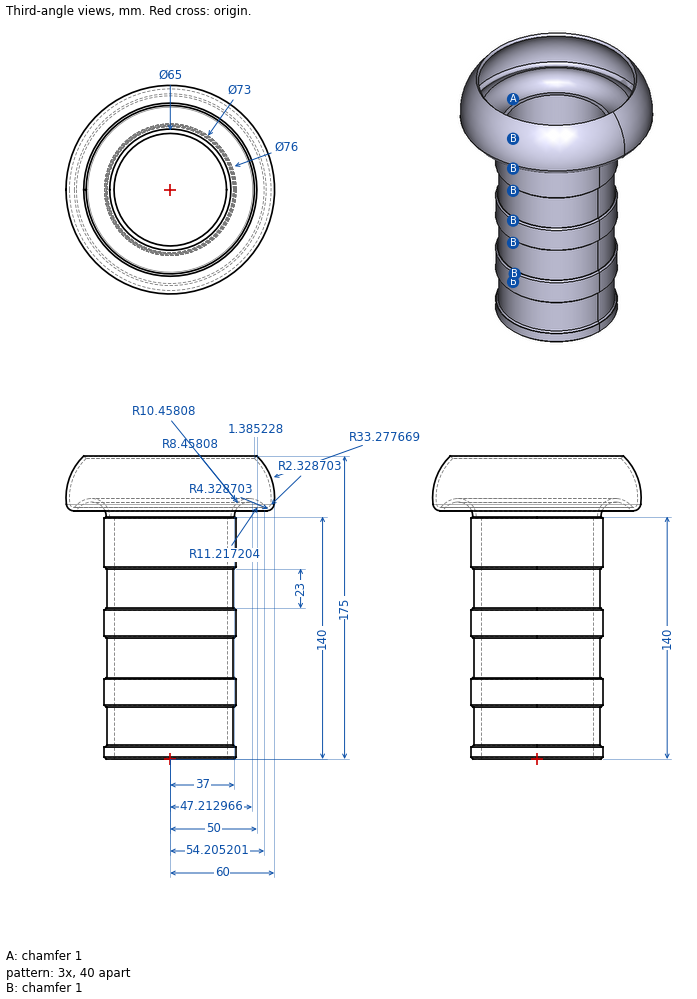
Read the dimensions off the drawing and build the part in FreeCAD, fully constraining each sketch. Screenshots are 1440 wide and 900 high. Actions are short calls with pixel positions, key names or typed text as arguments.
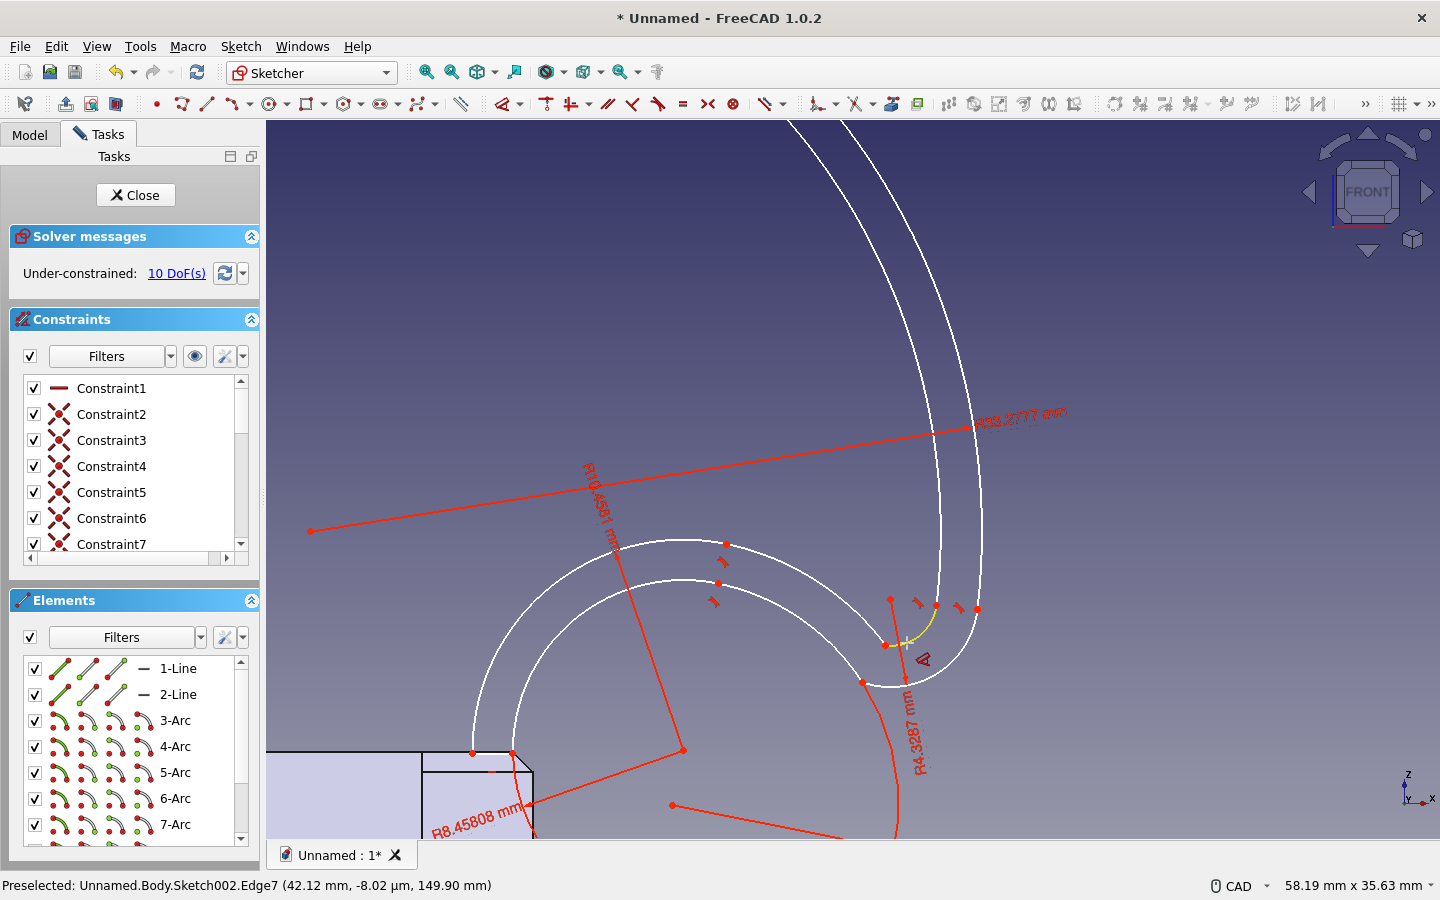
click(907, 643)
click(964, 572)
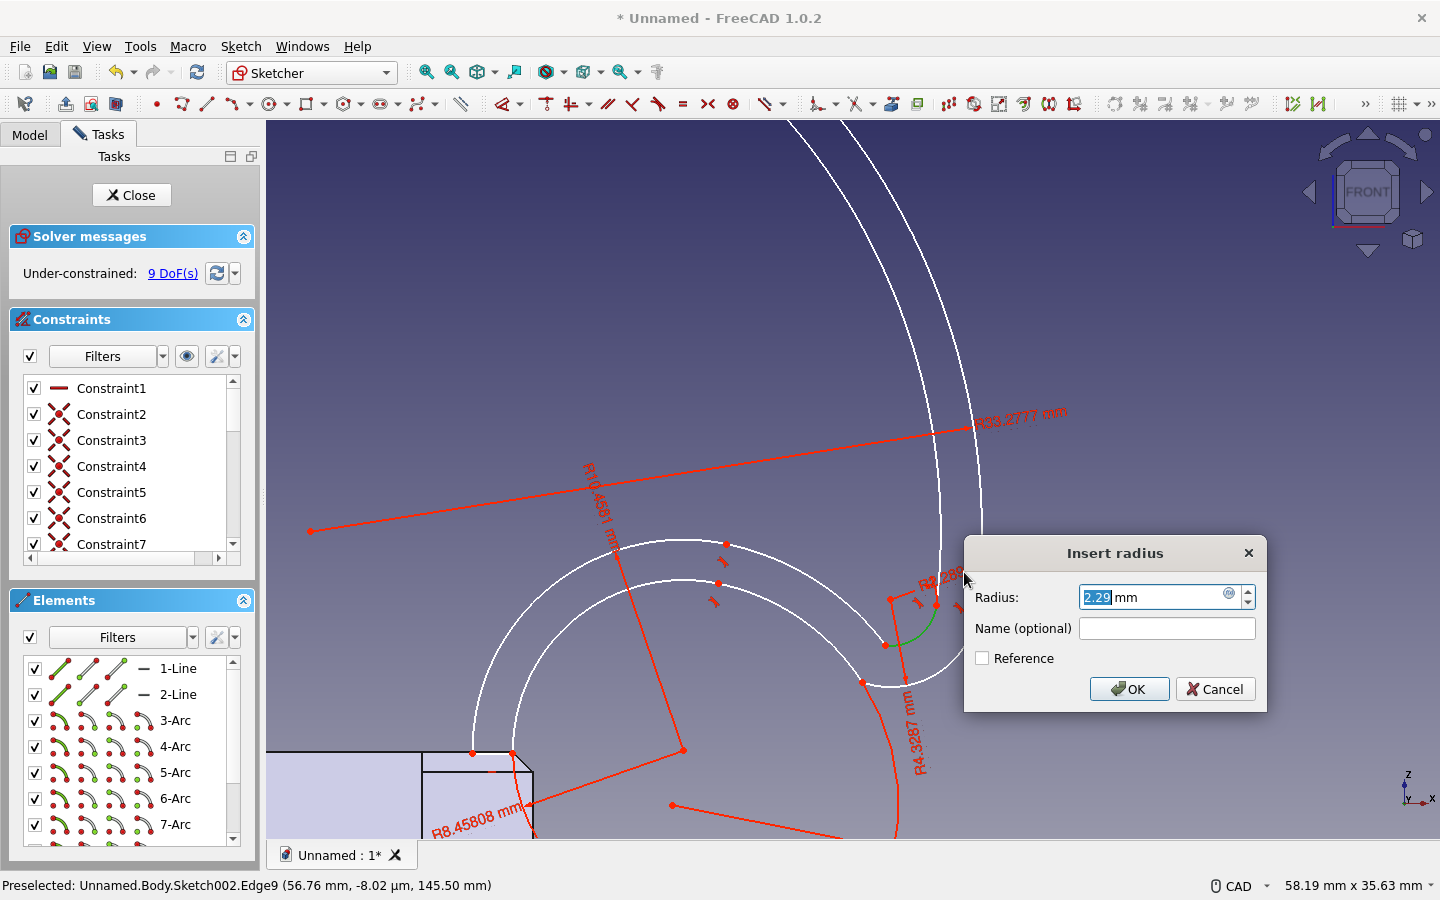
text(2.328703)
key(Return)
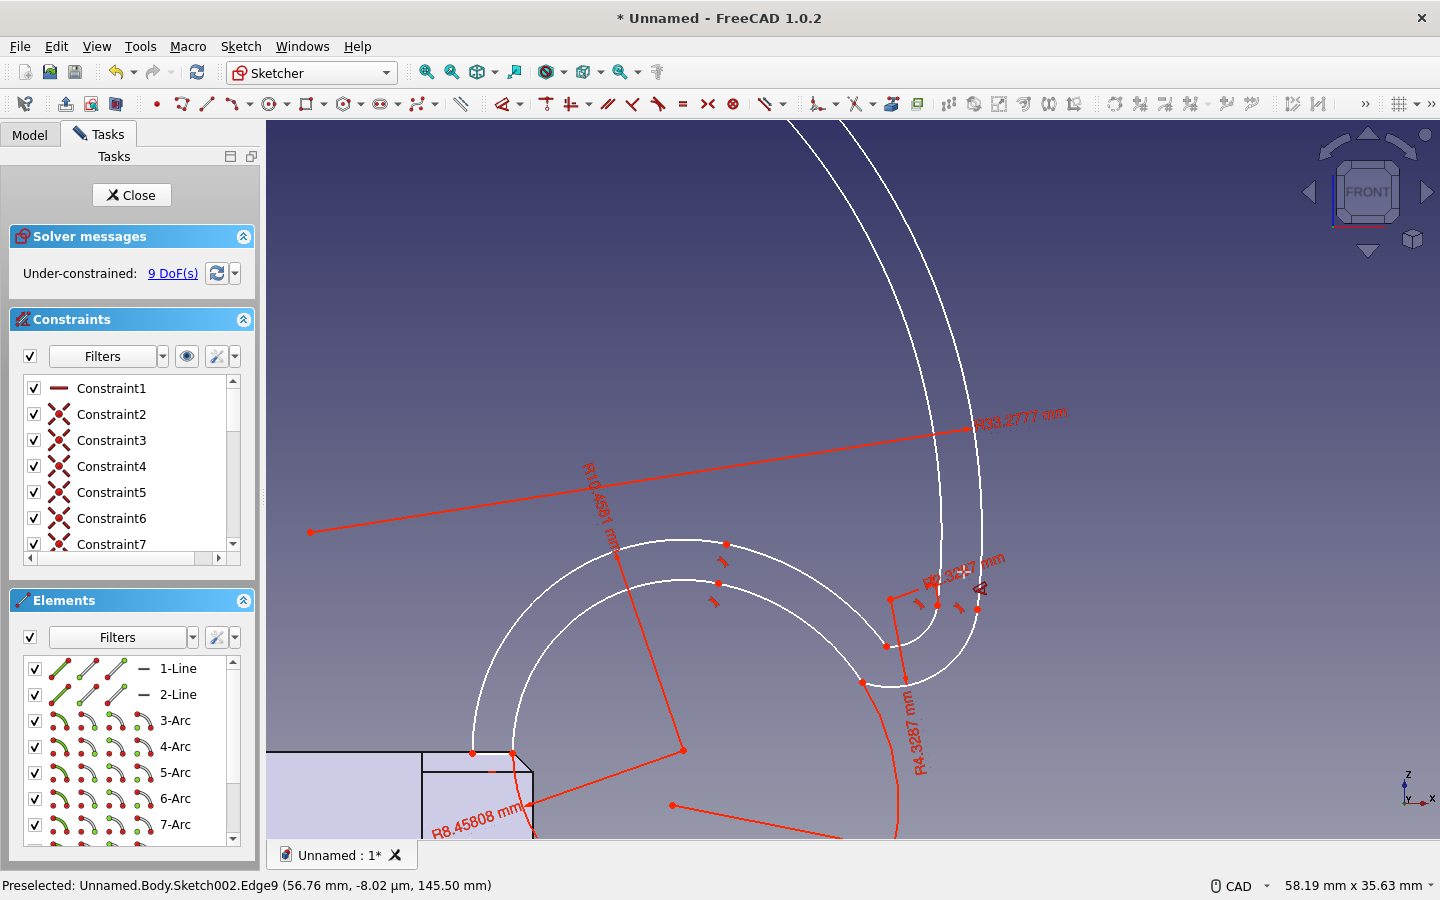
scroll(907, 643, down, 2)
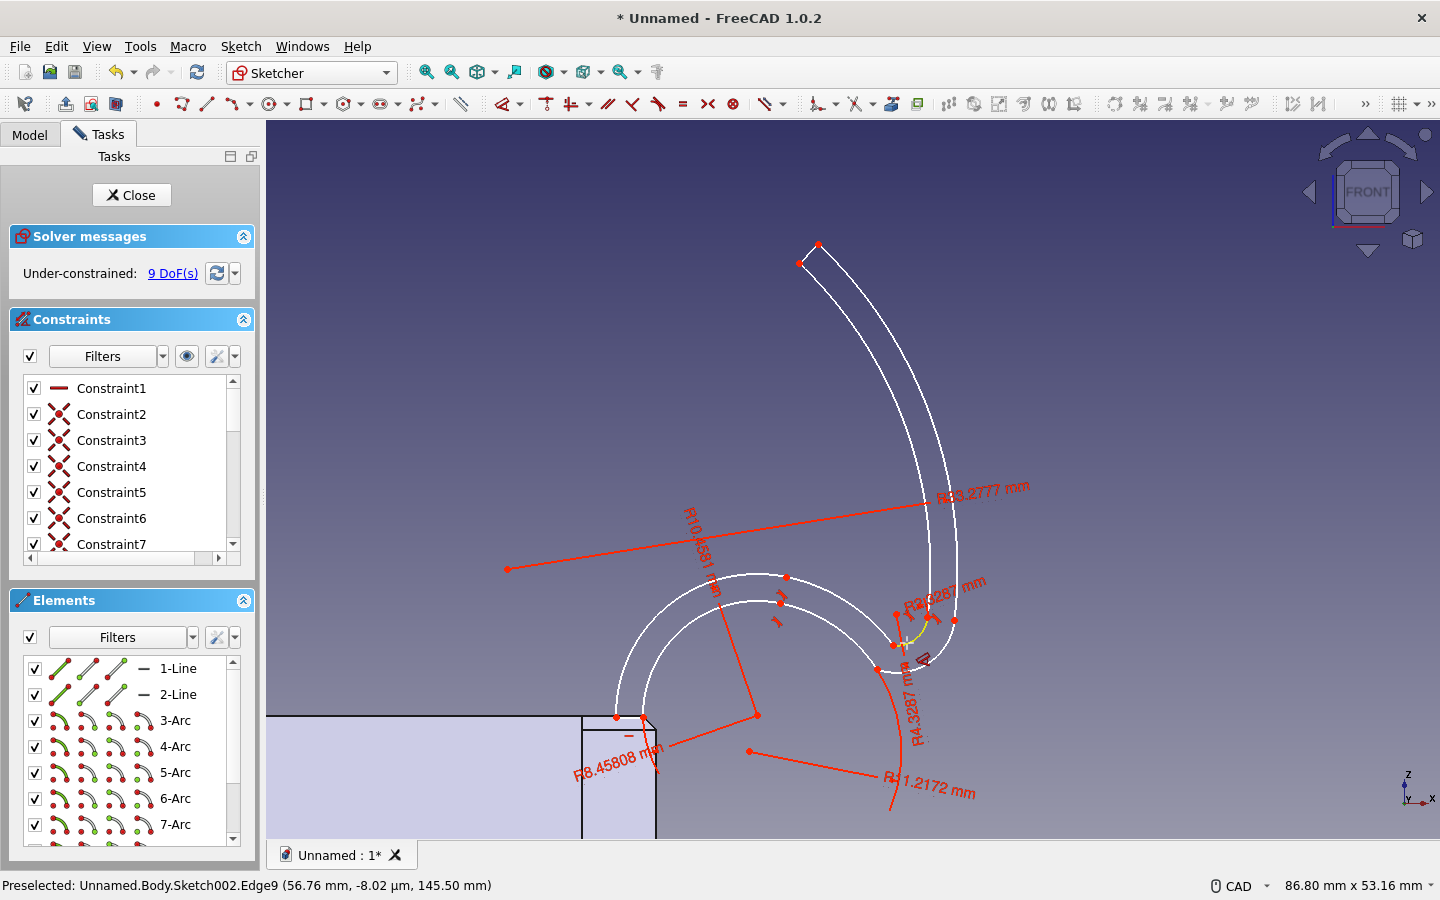
click(819, 244)
click(556, 210)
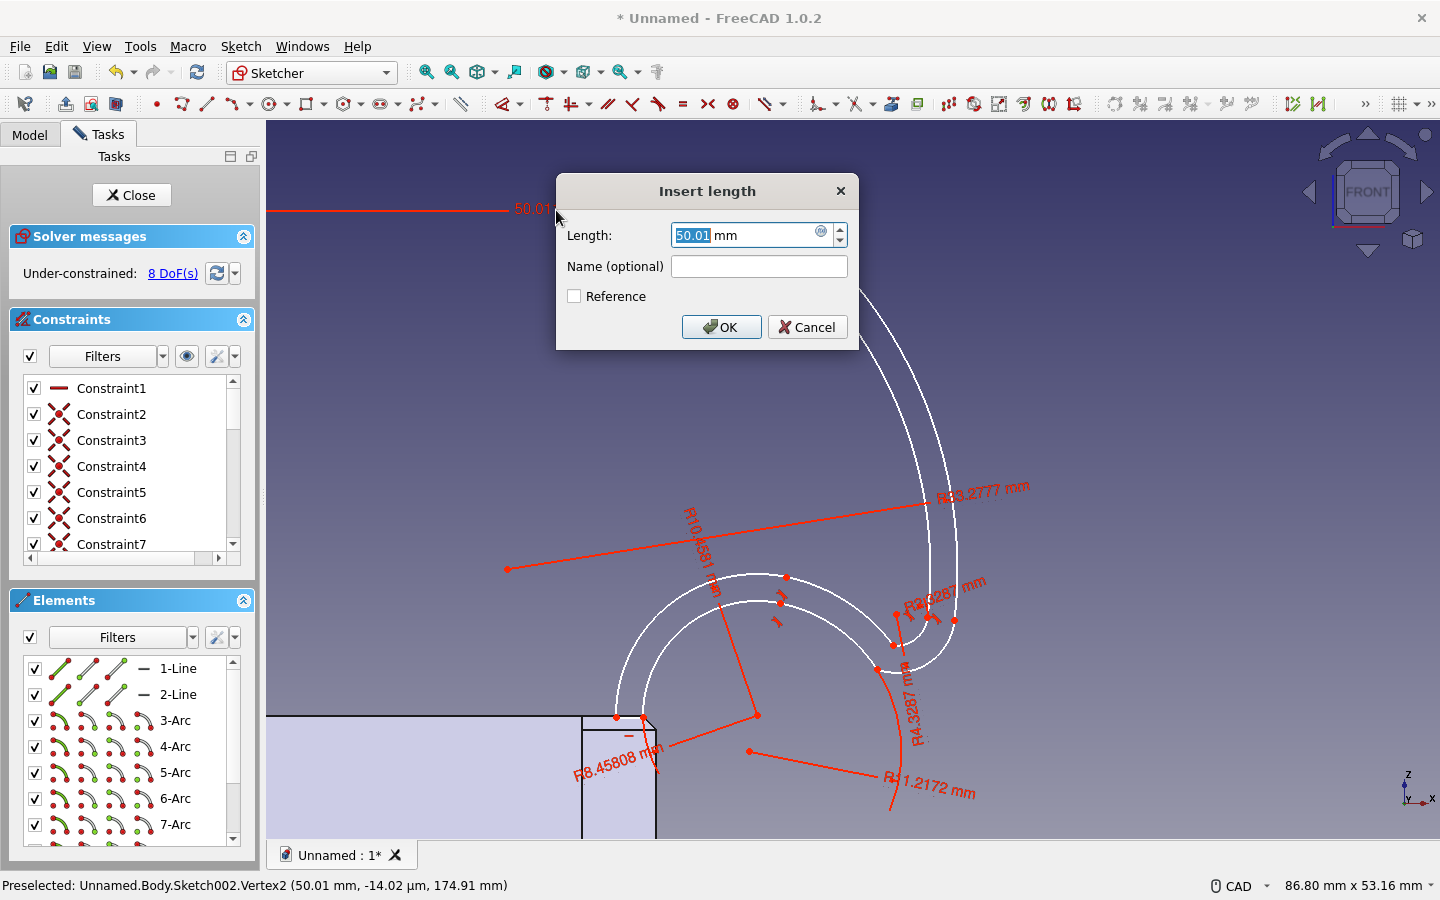
text(50)
key(Return)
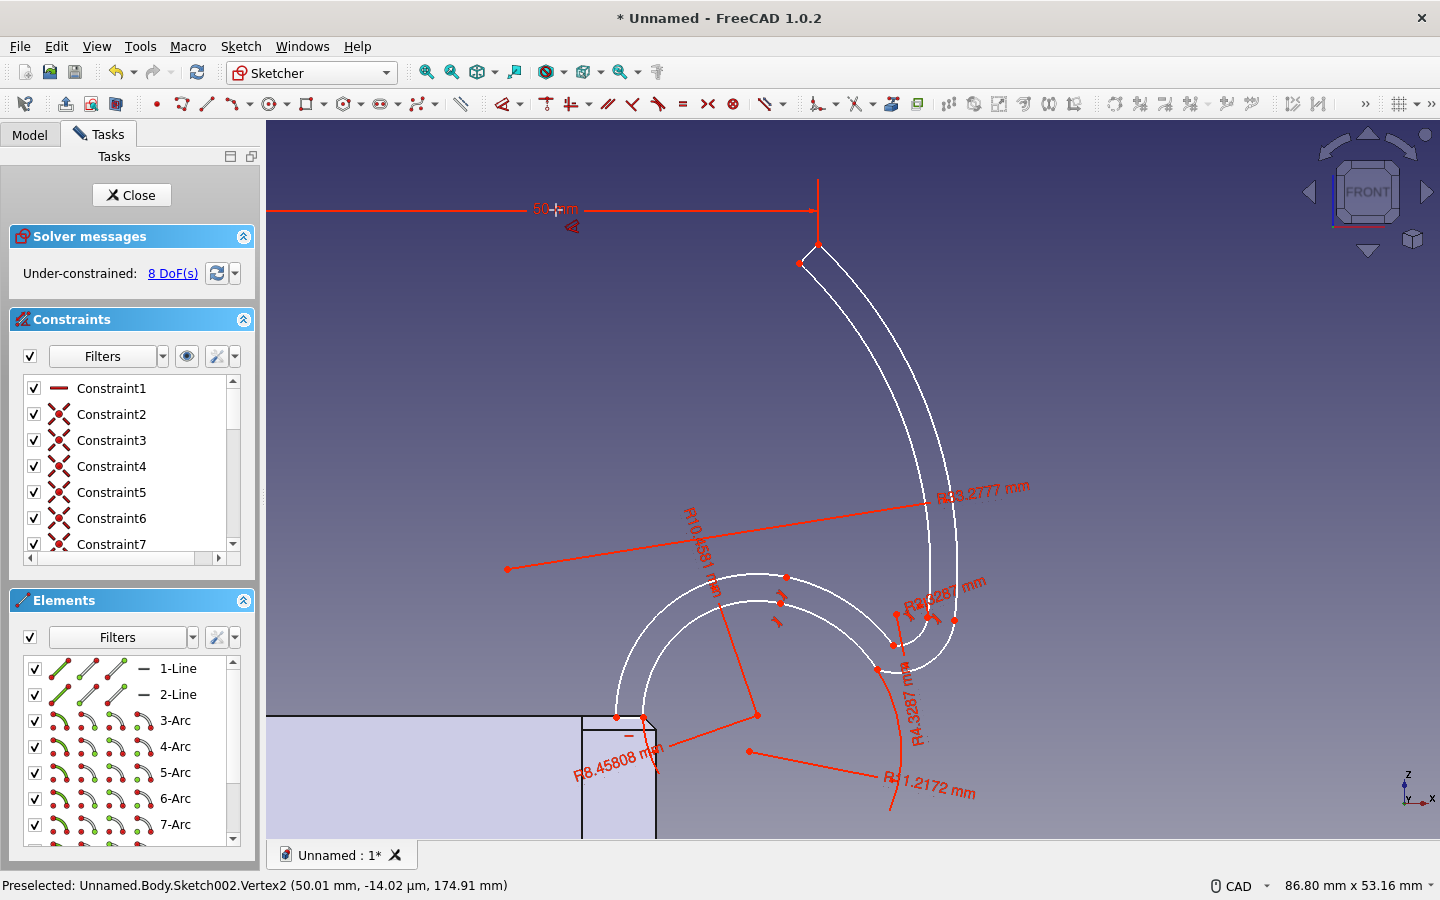
click(643, 718)
click(469, 684)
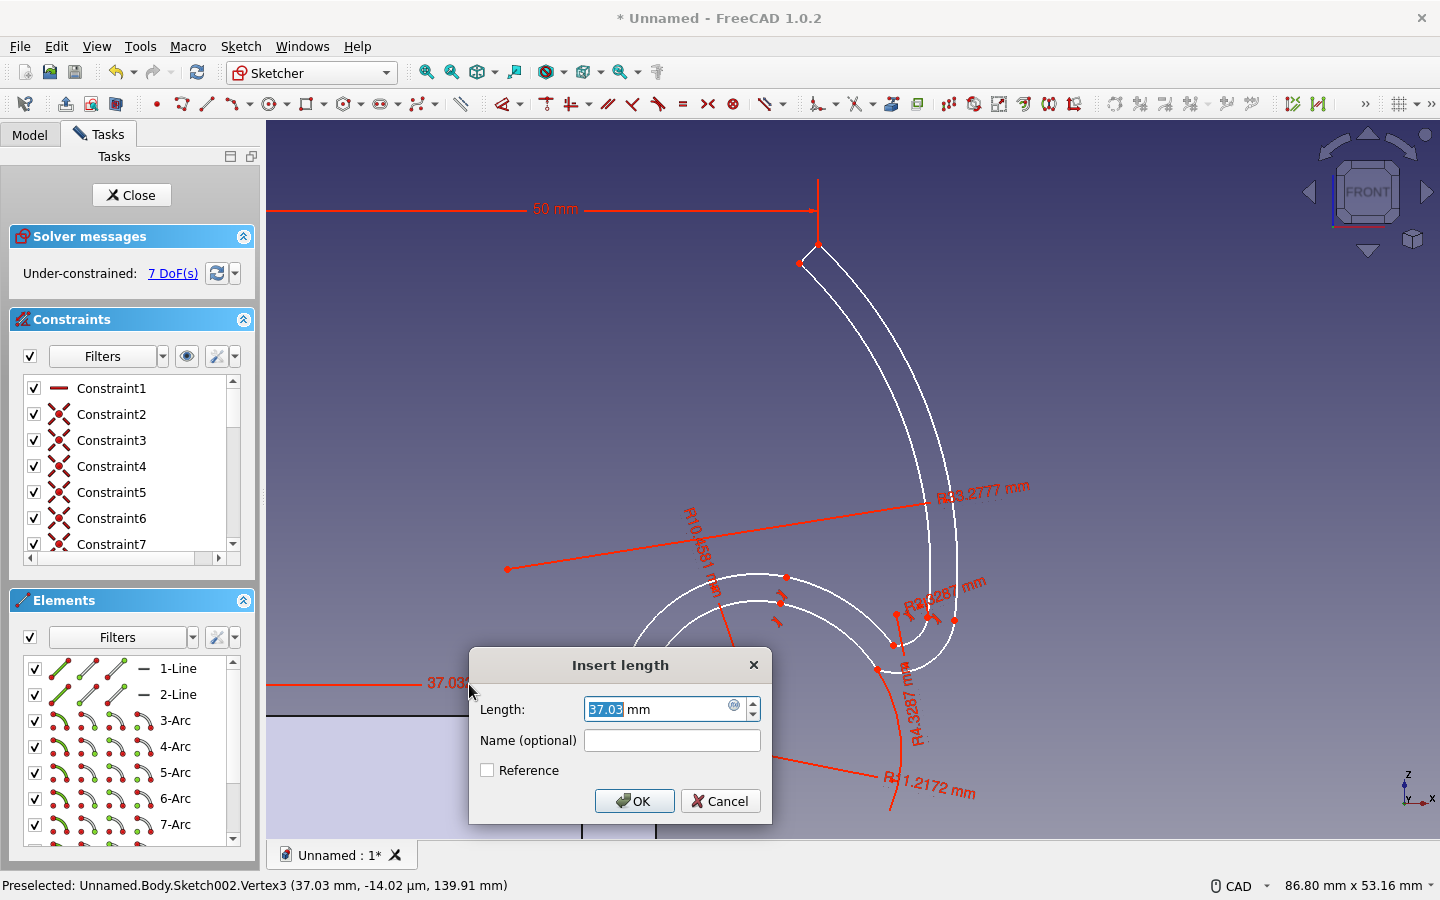
text(37)
key(Return)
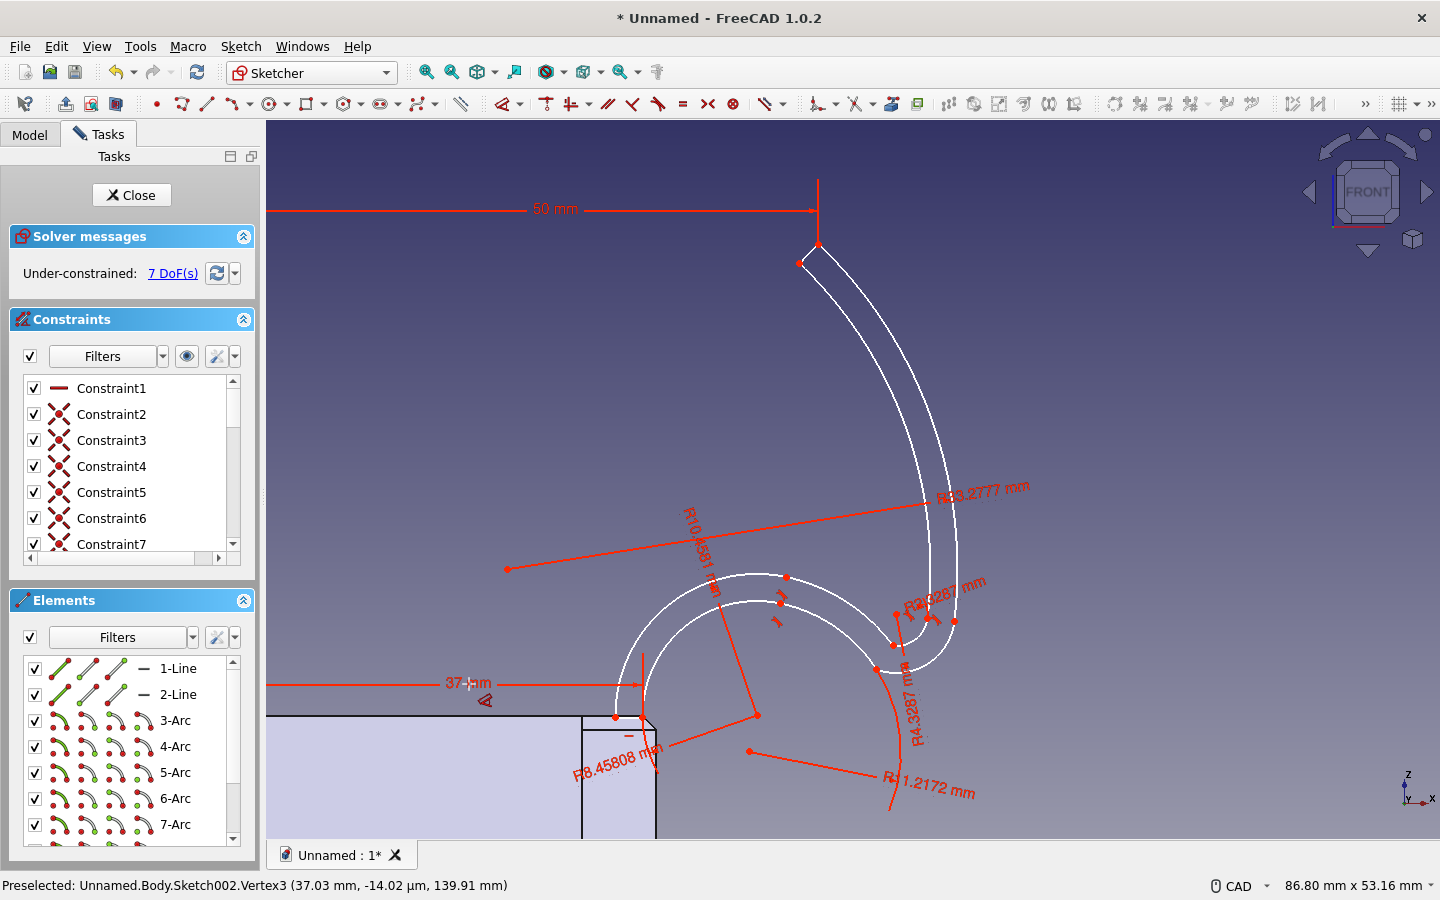
click(954, 621)
click(624, 587)